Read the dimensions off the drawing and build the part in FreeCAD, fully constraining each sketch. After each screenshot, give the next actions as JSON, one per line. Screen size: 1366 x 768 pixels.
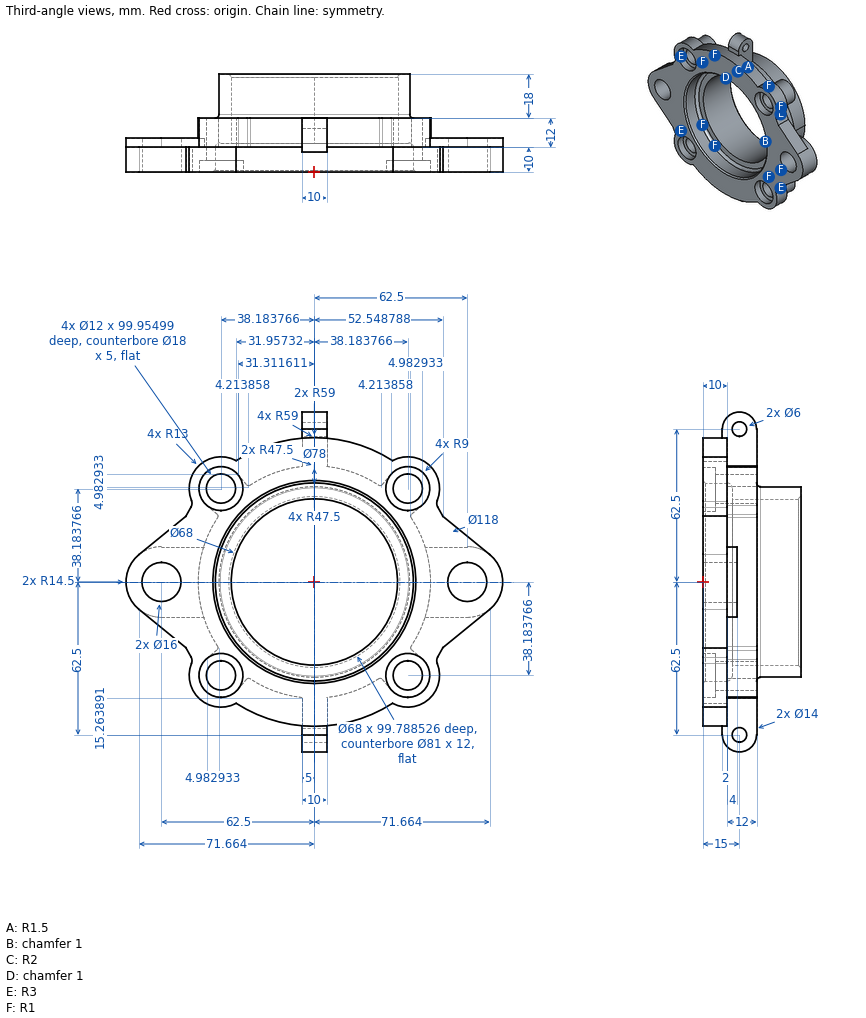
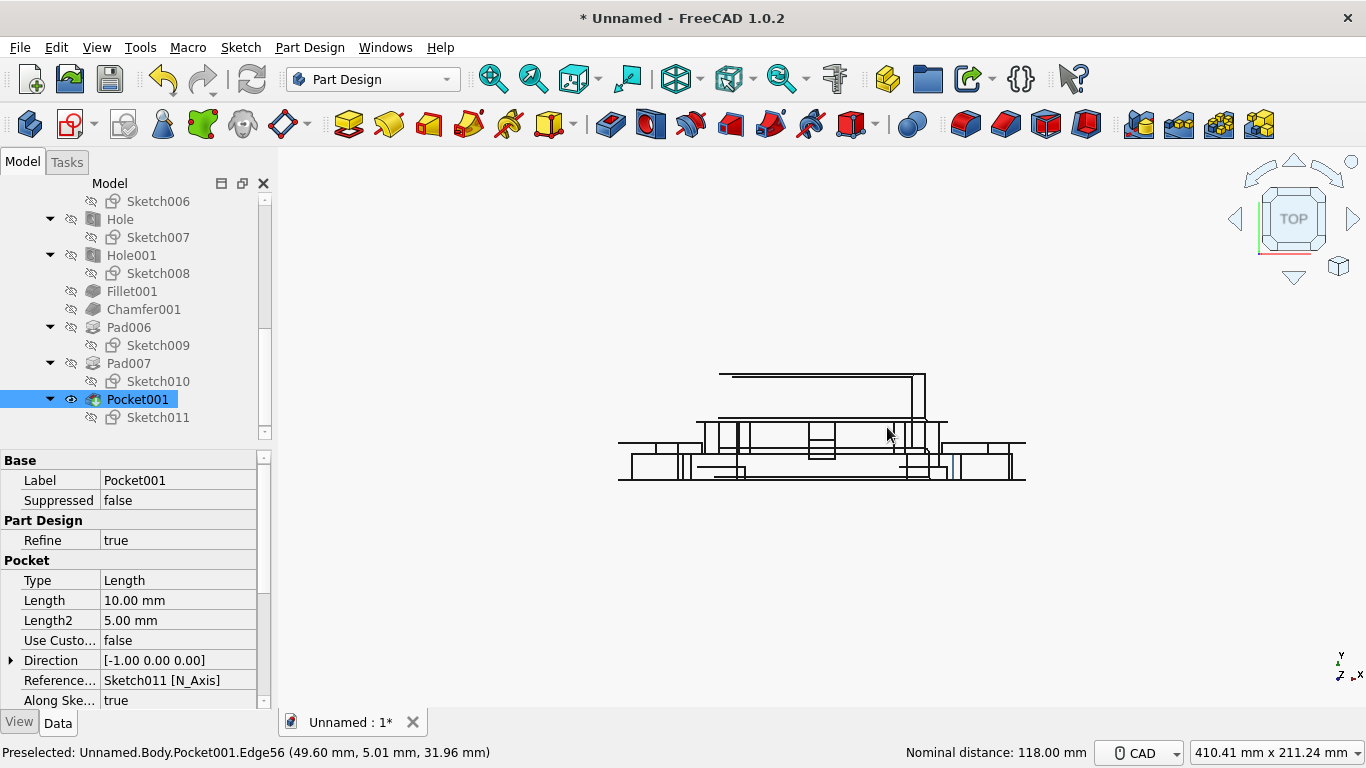
{"action": "left_click", "coordinate": [494, 80]}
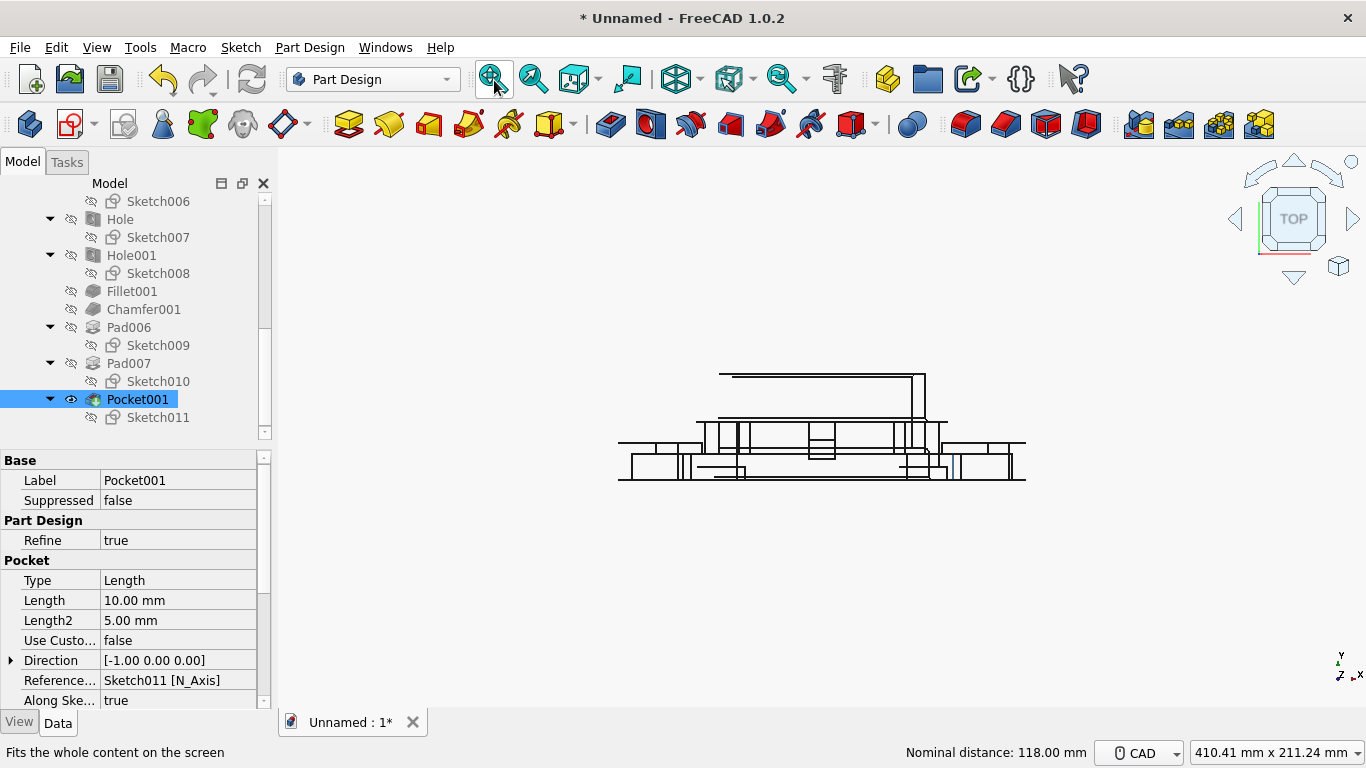
{"action": "left_click", "coordinate": [691, 466], "text": "ctrl"}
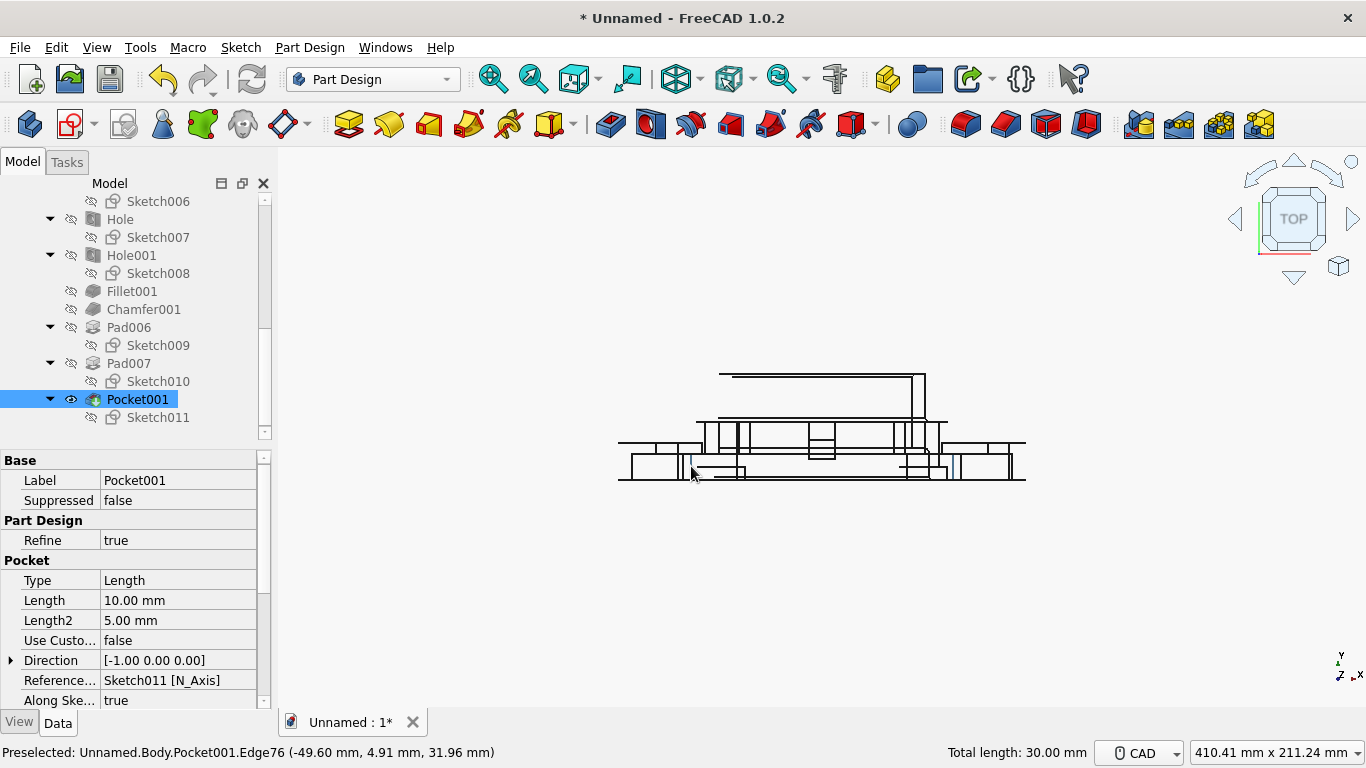
{"action": "key", "text": "1"}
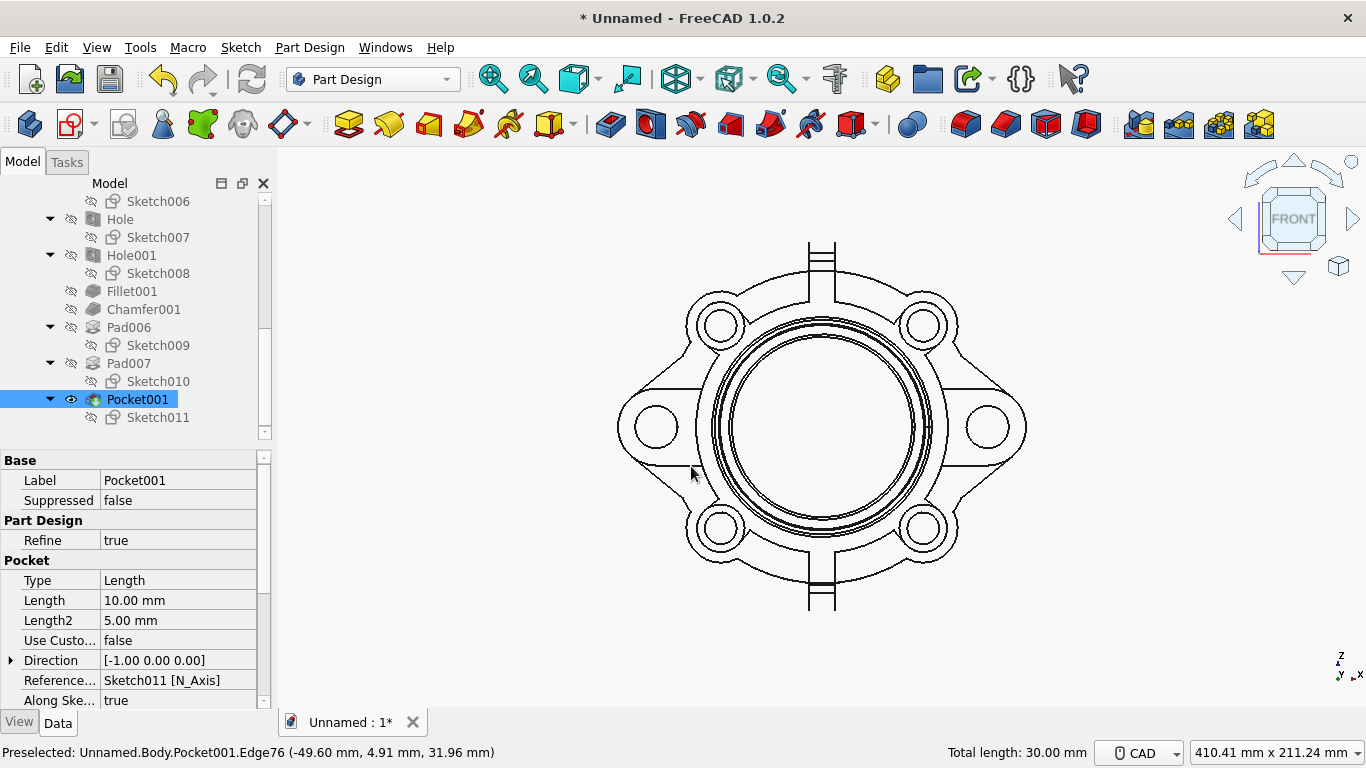
{"action": "key", "text": "3"}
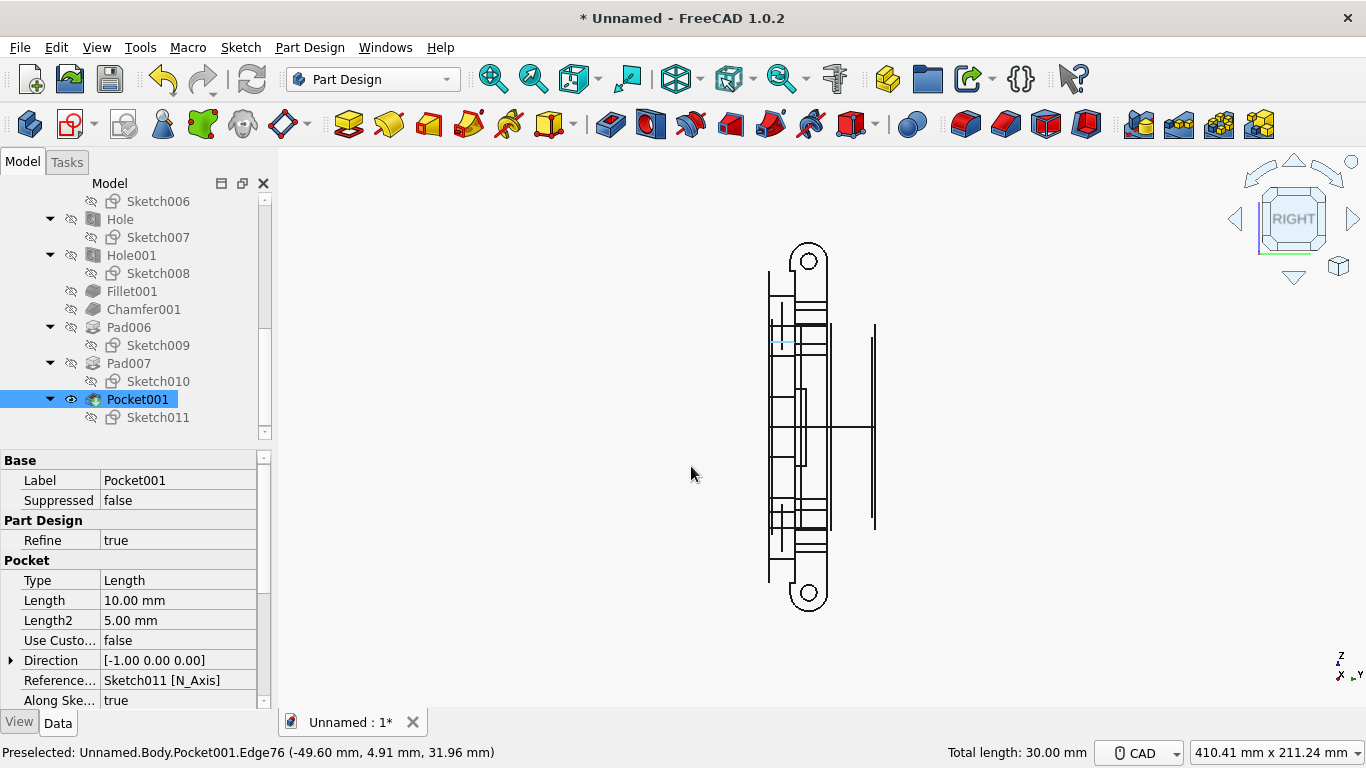
{"action": "left_click", "coordinate": [782, 511], "text": "ctrl"}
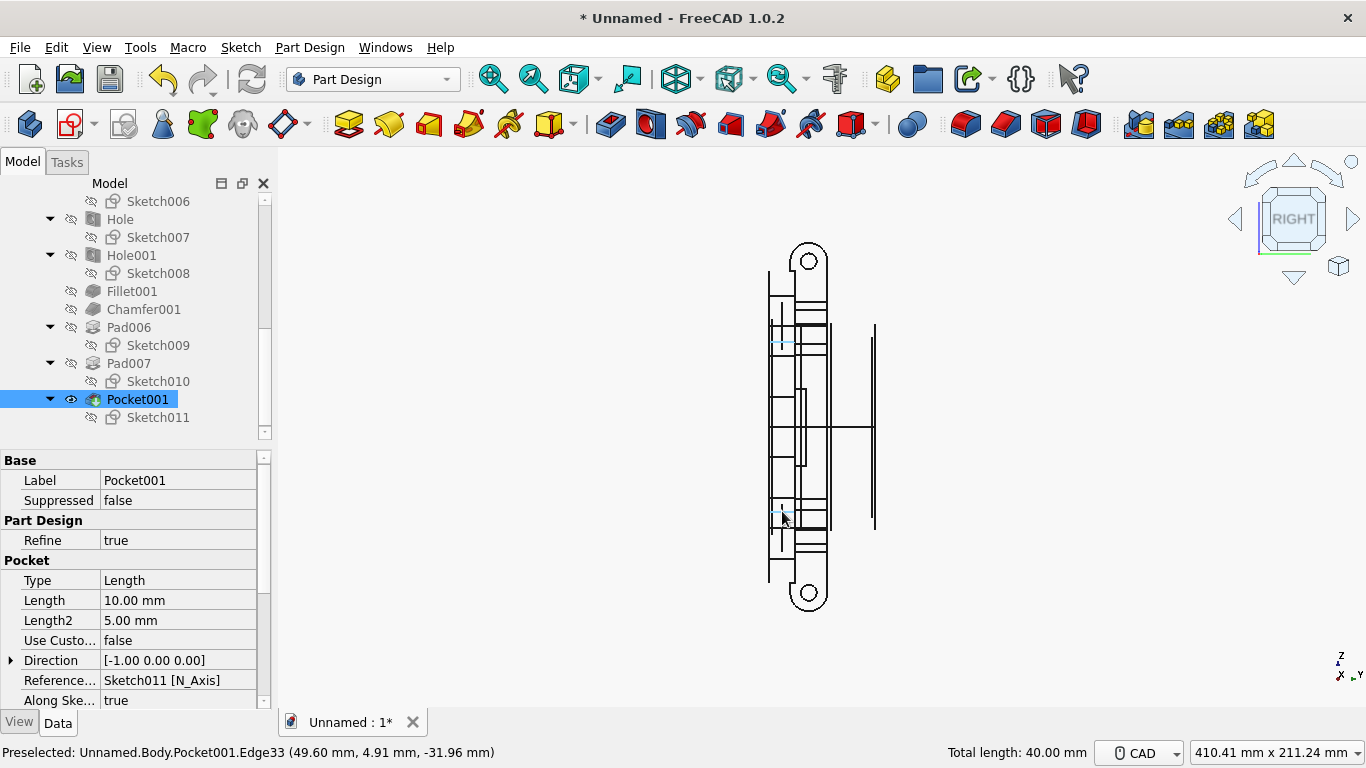
{"action": "key", "text": "v 1"}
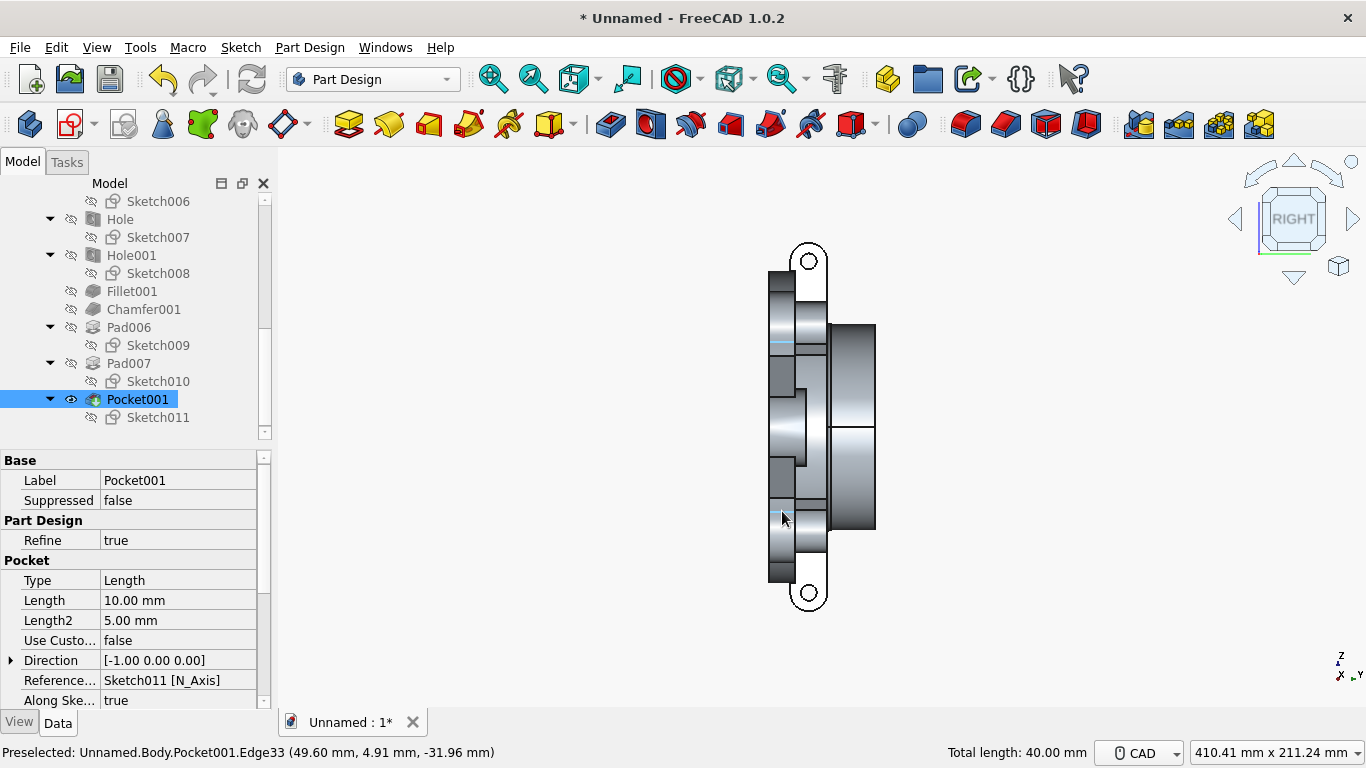
{"action": "left_click", "coordinate": [966, 124]}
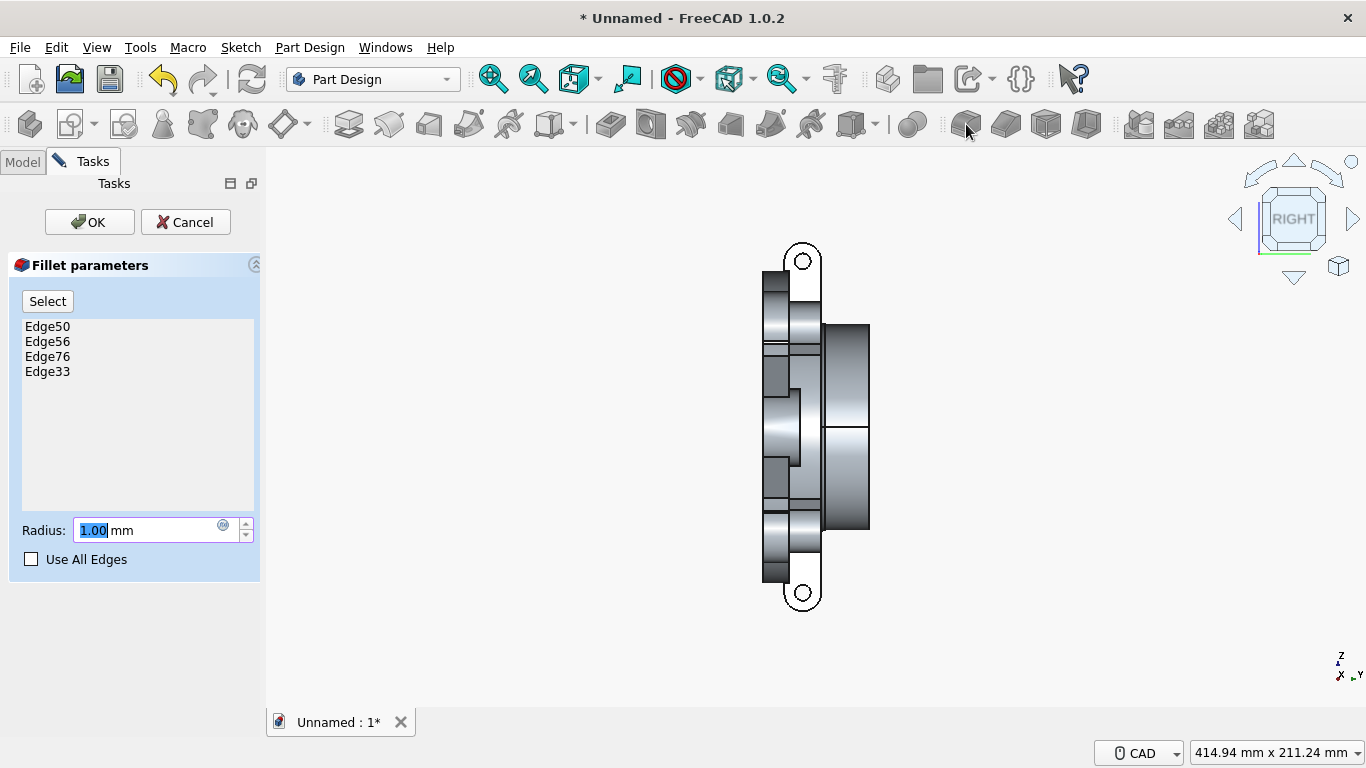
{"action": "type", "text": "3"}
{"action": "key", "text": "Tab"}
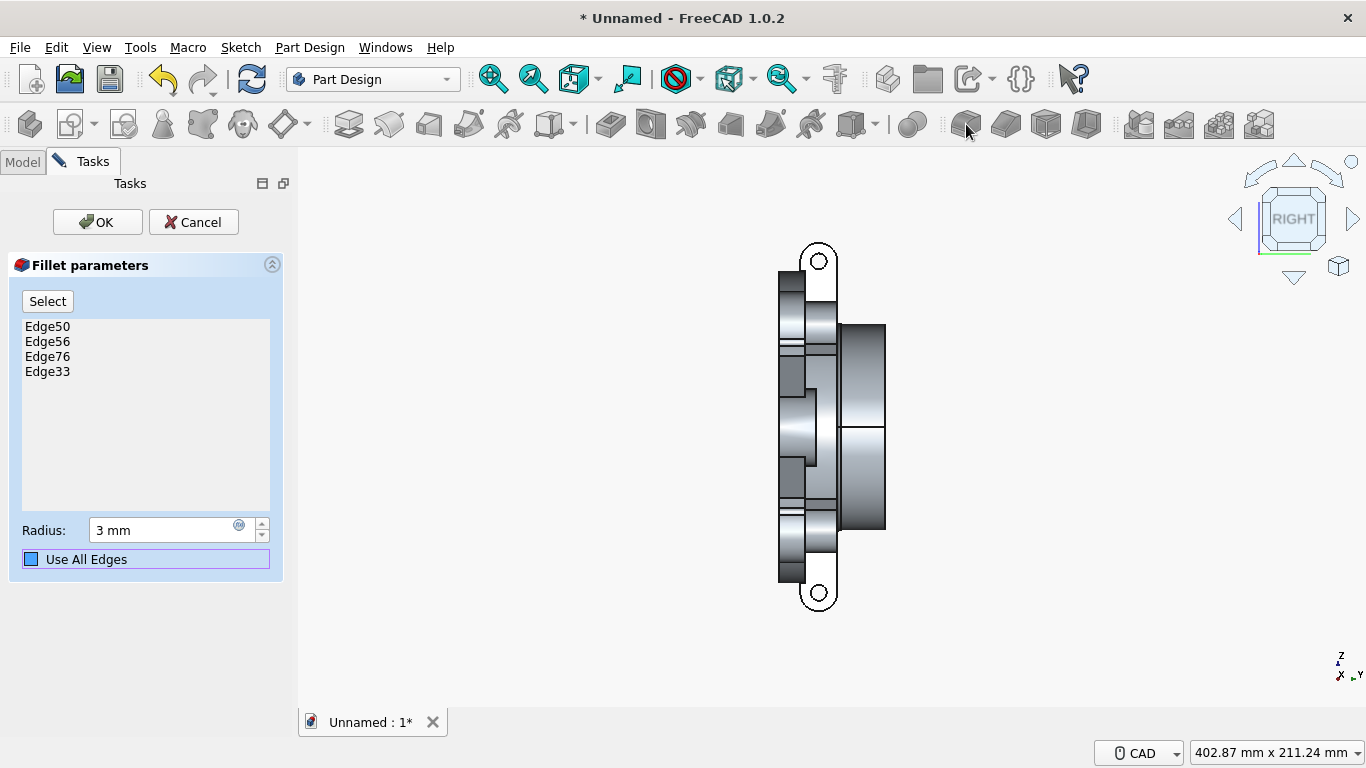
{"action": "left_click", "coordinate": [98, 222]}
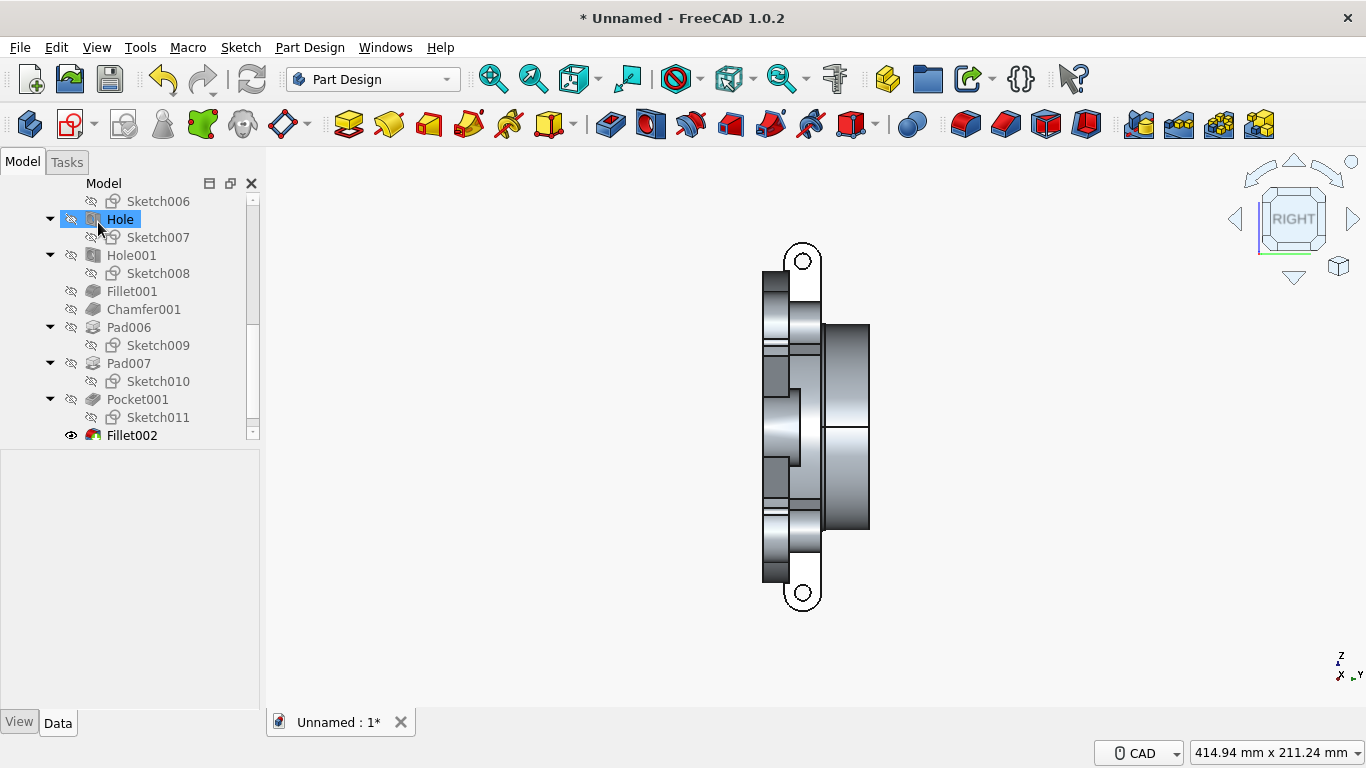
{"action": "key", "text": "0"}